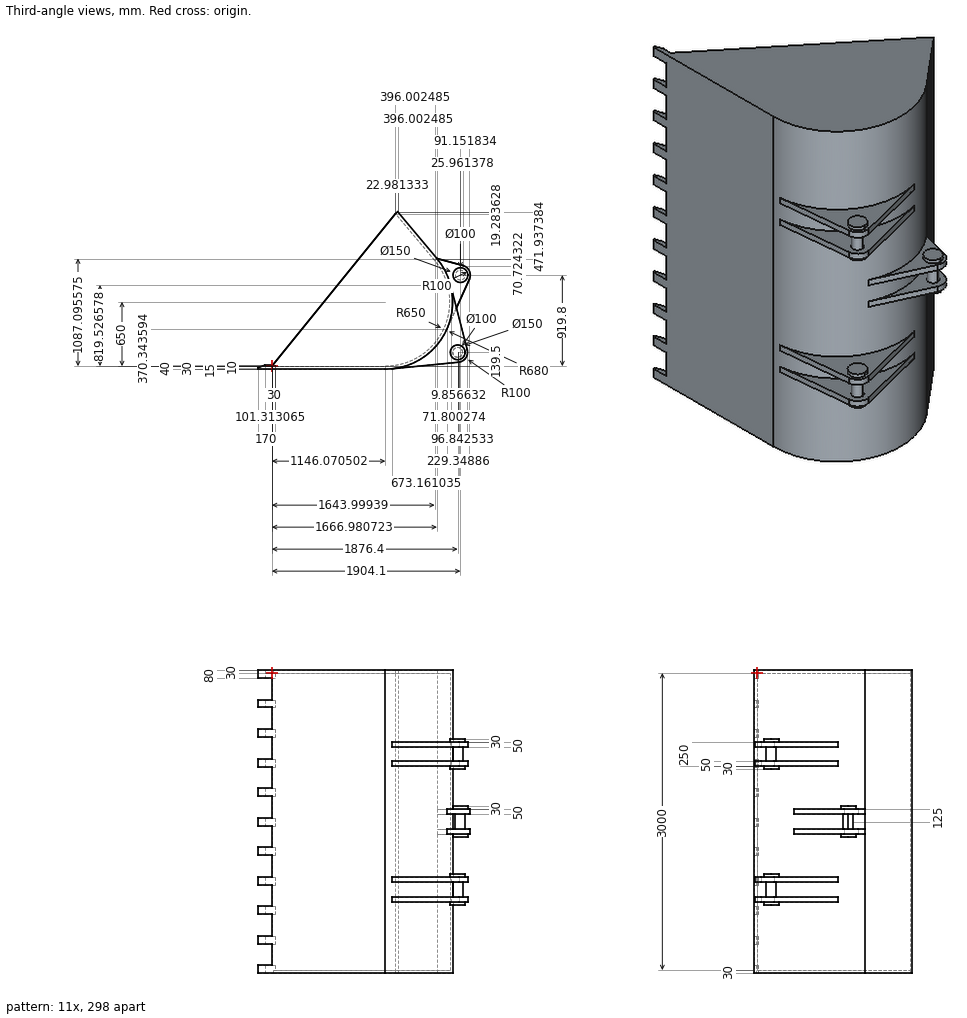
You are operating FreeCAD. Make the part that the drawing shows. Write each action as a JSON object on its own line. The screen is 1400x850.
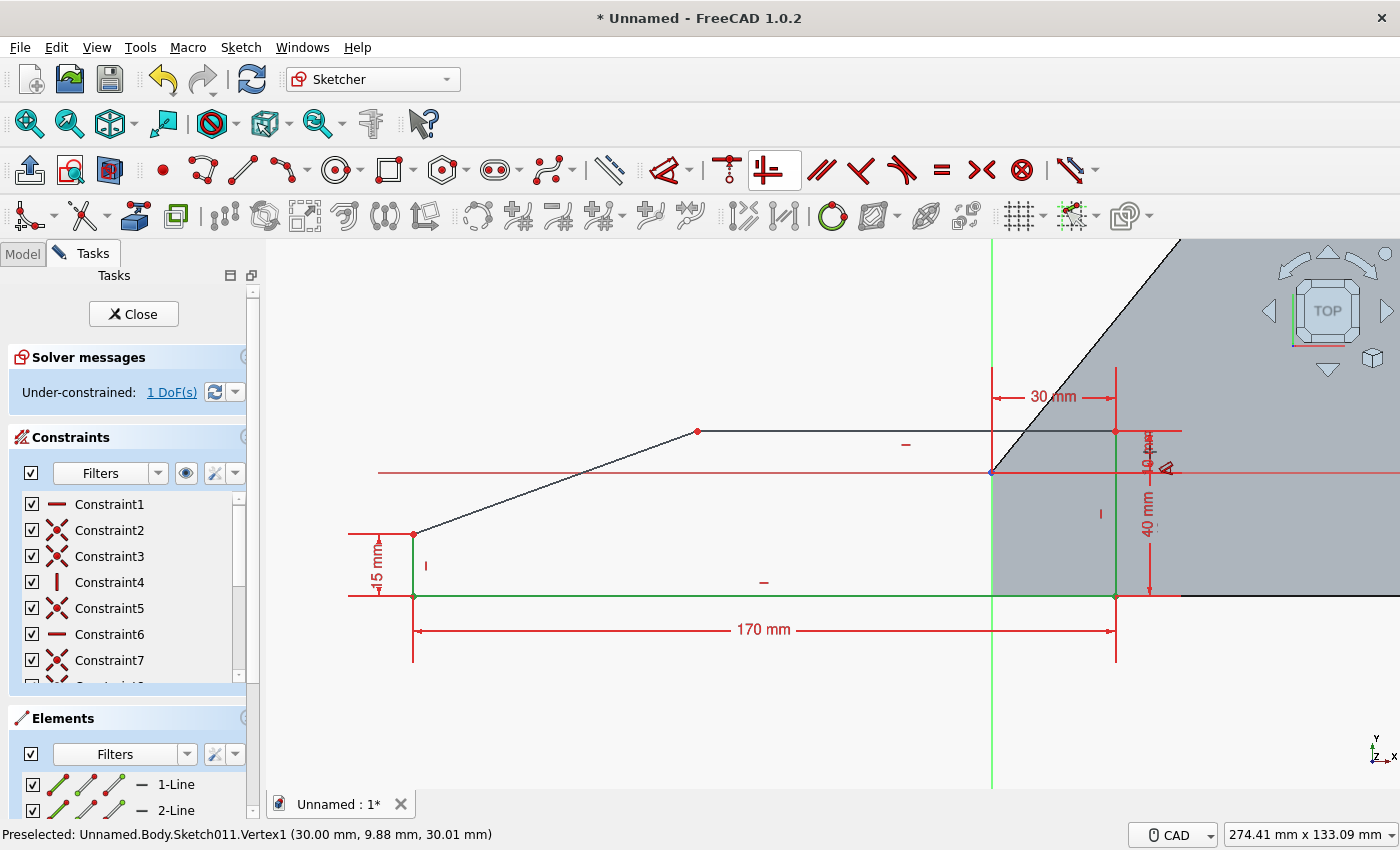
{"action": "left_click", "coordinate": [990, 431]}
{"action": "left_click", "coordinate": [906, 397]}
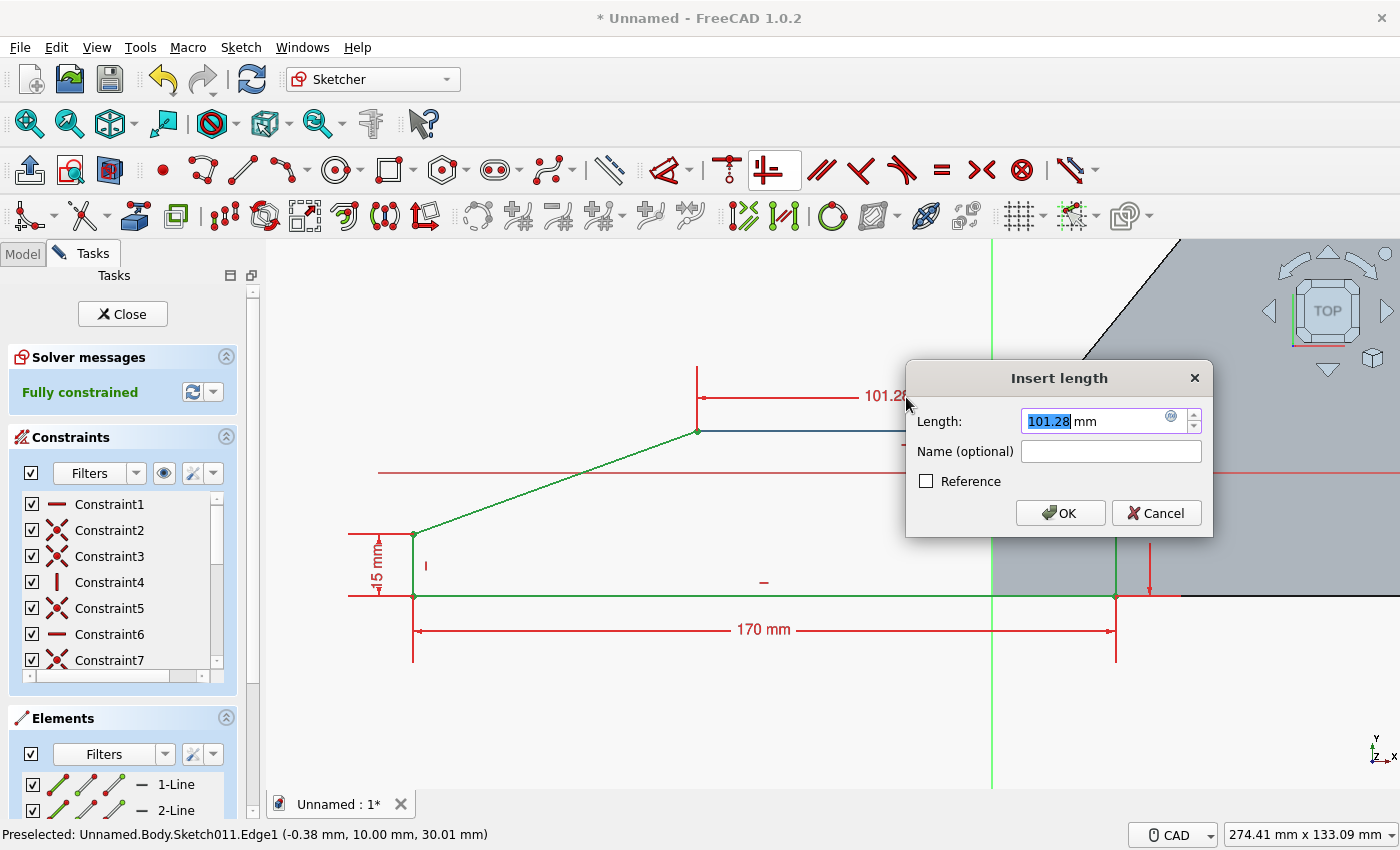
{"action": "type", "text": "101.313065"}
{"action": "key", "text": "Return"}
{"action": "key", "text": "Escape"}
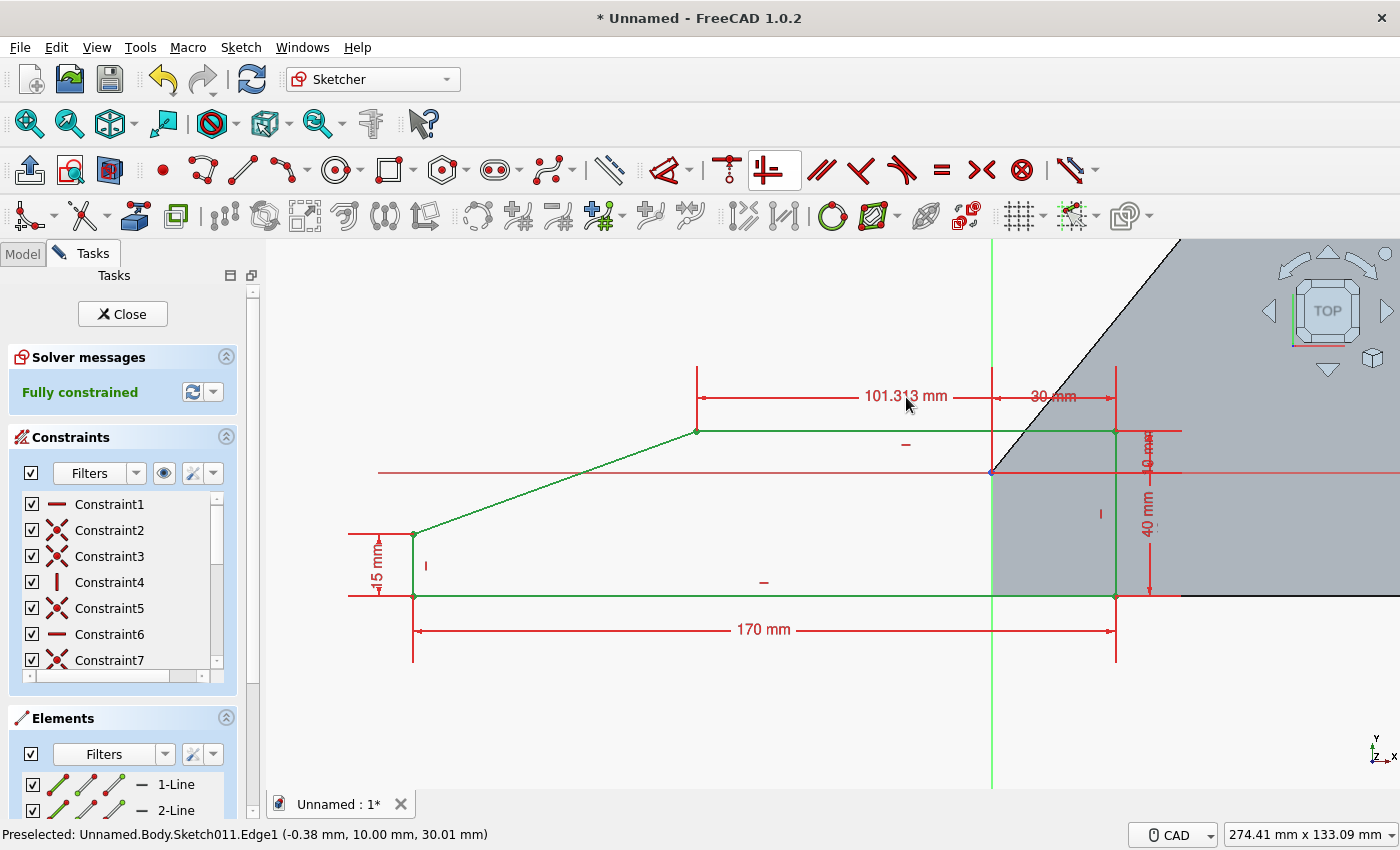
{"action": "left_click", "coordinate": [123, 314]}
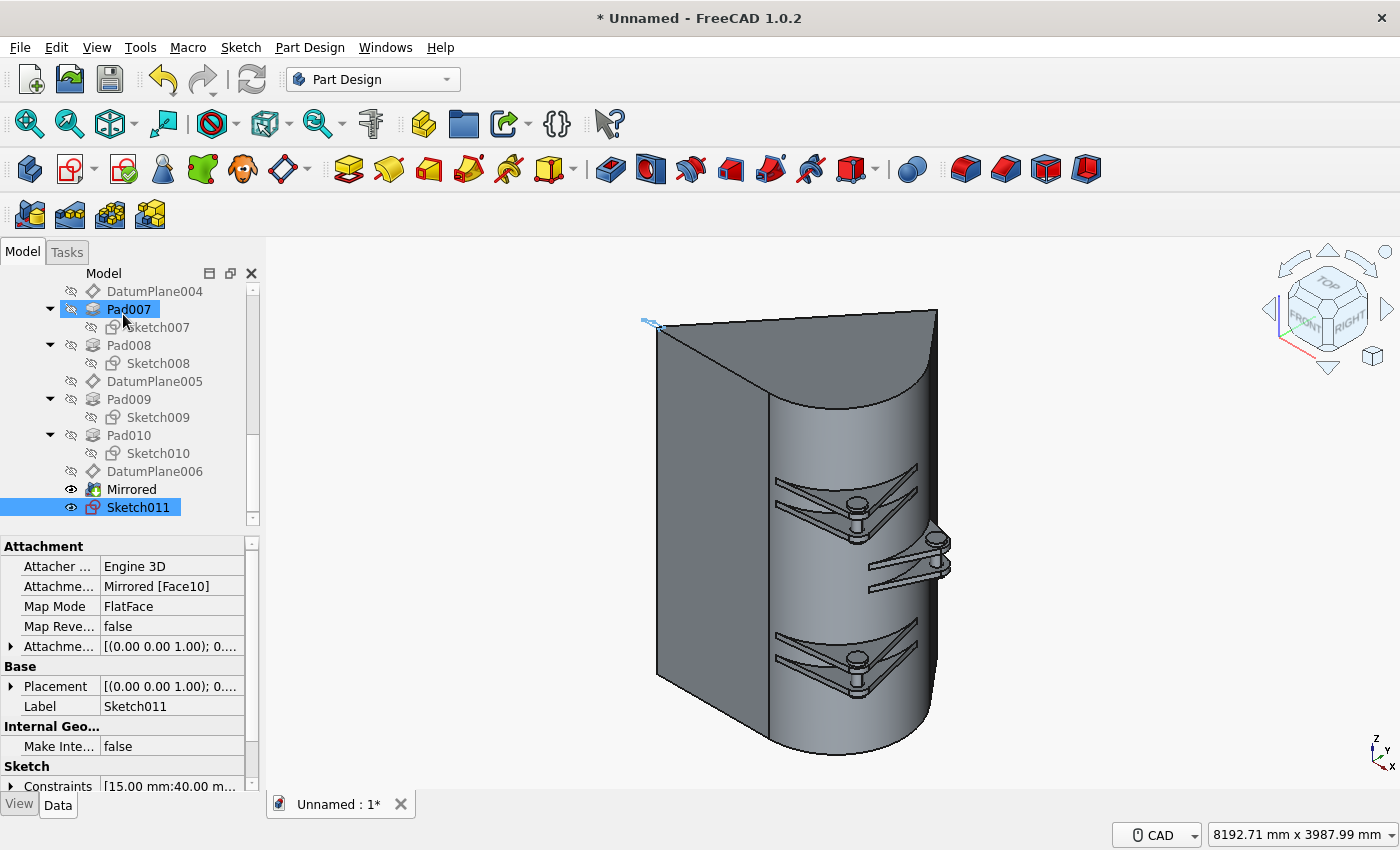
{"action": "left_click", "coordinate": [350, 170]}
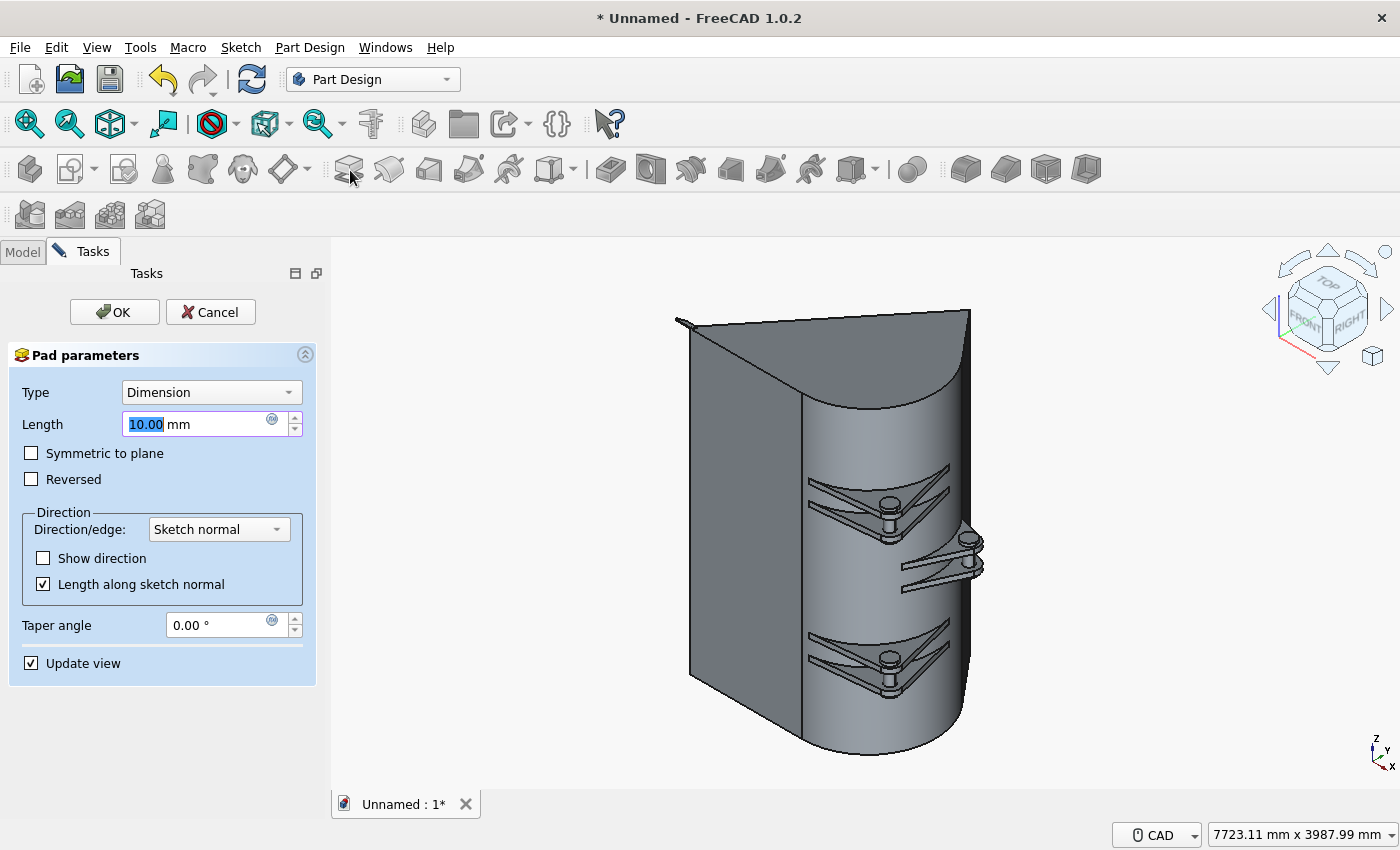
{"action": "type", "text": "80"}
{"action": "key", "text": "Tab"}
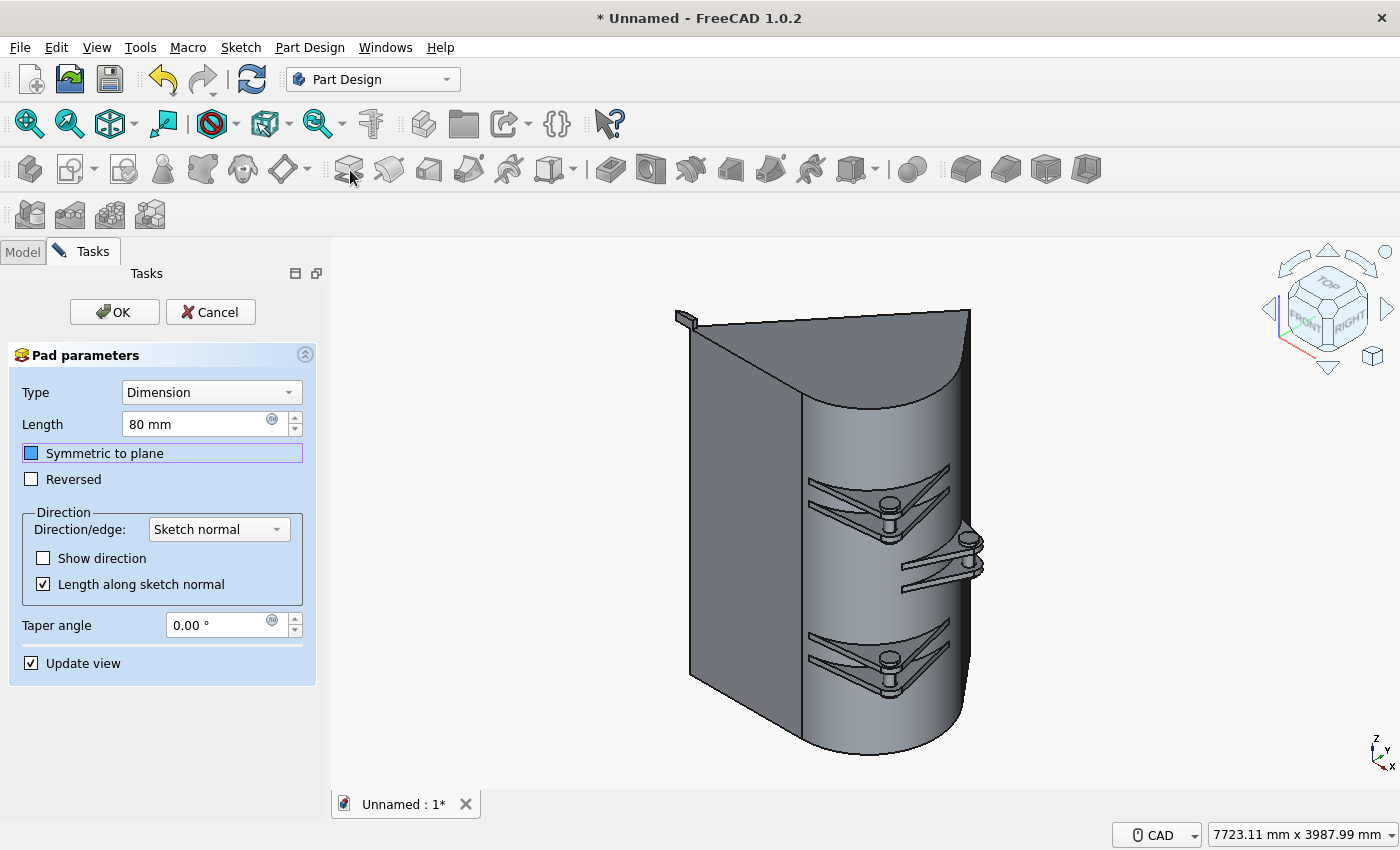
{"action": "left_click", "coordinate": [30, 479]}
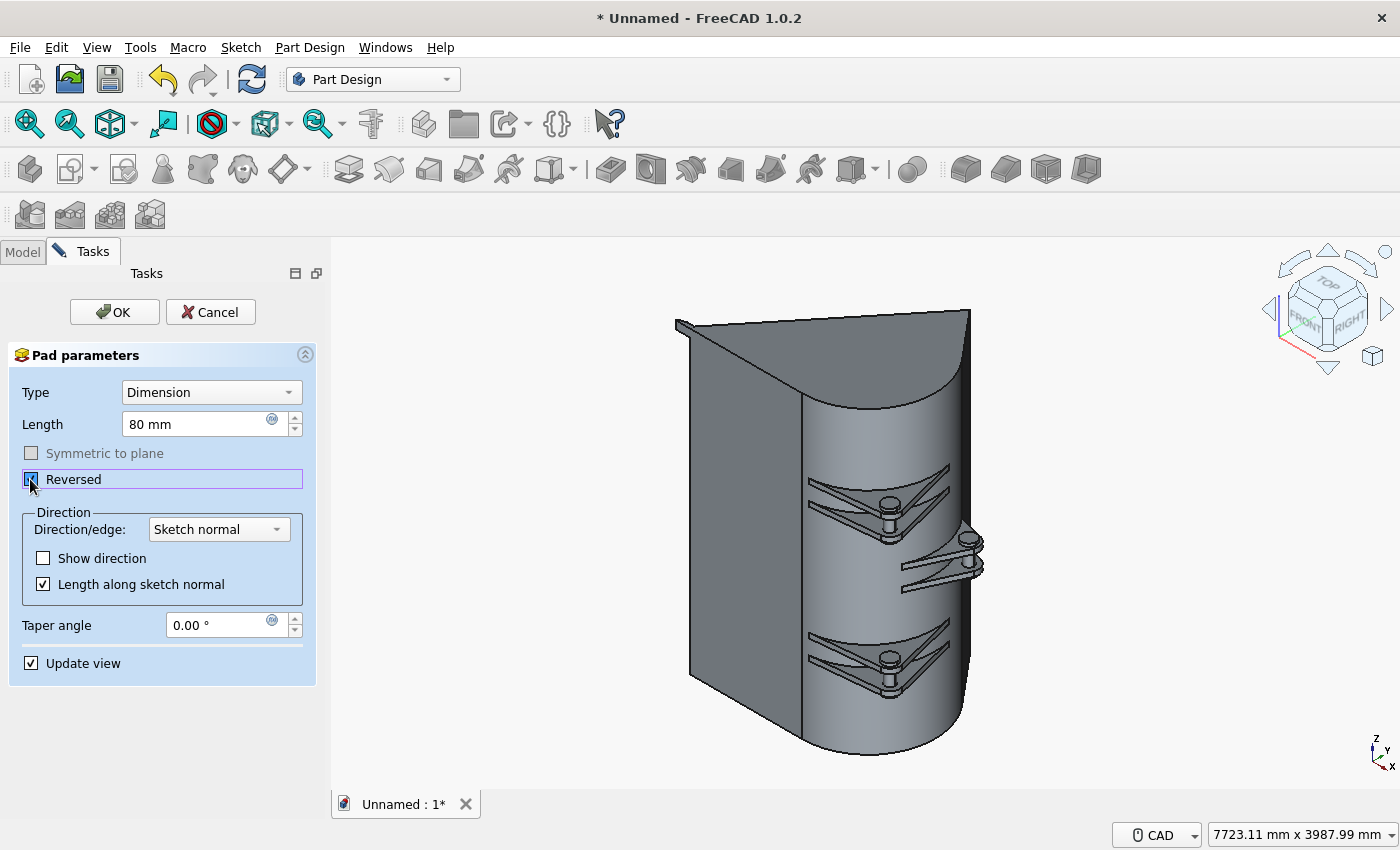
{"action": "left_click", "coordinate": [115, 312]}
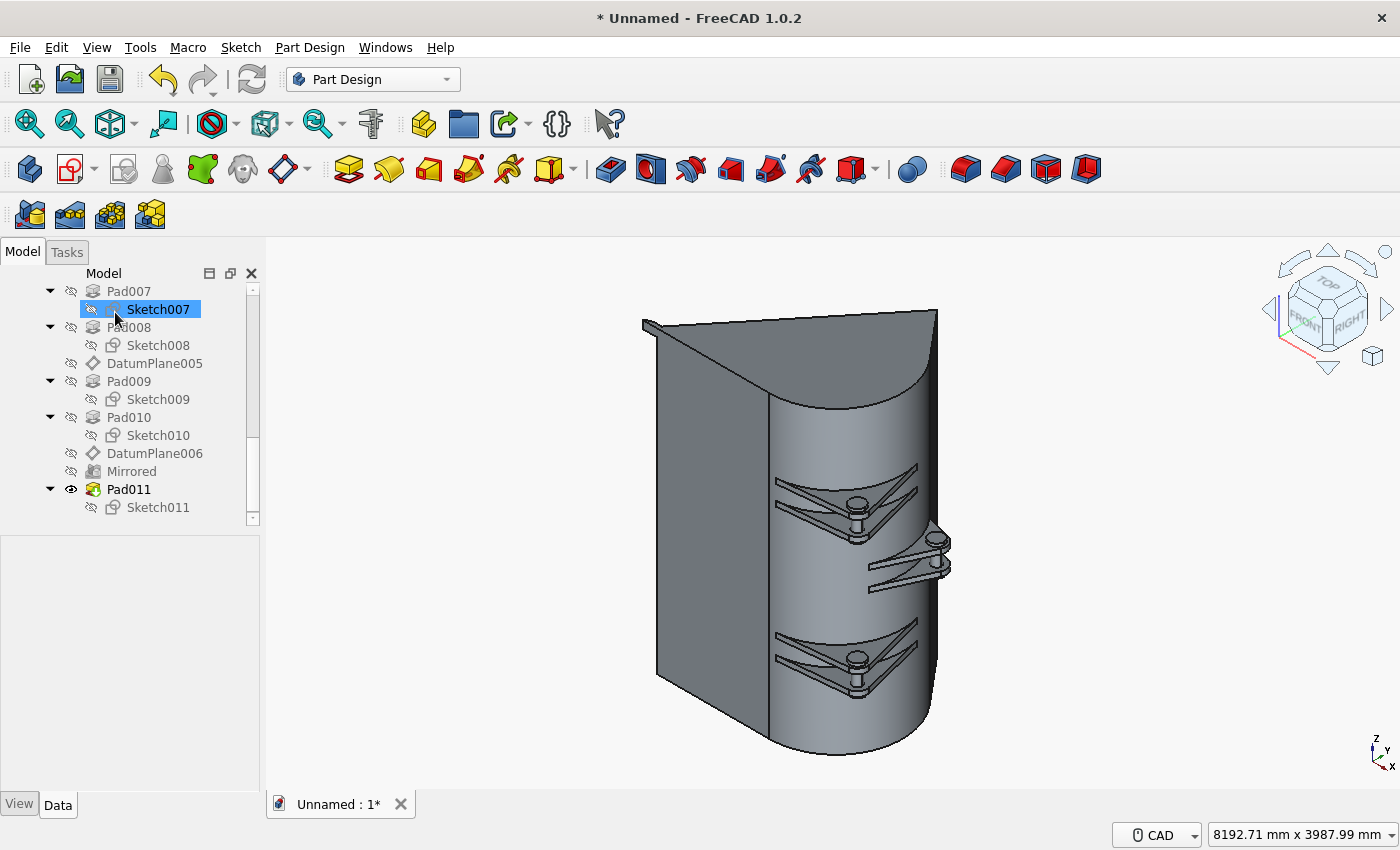
{"action": "left_click", "coordinate": [30, 124]}